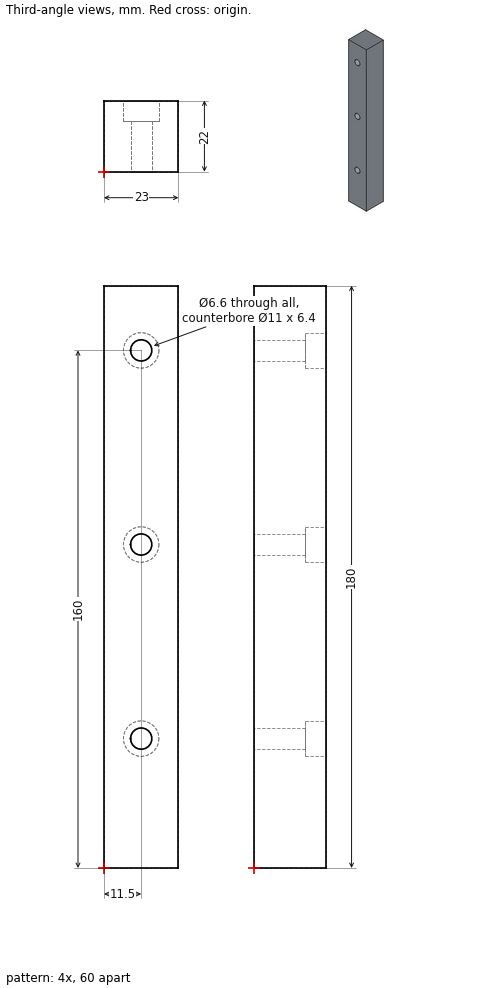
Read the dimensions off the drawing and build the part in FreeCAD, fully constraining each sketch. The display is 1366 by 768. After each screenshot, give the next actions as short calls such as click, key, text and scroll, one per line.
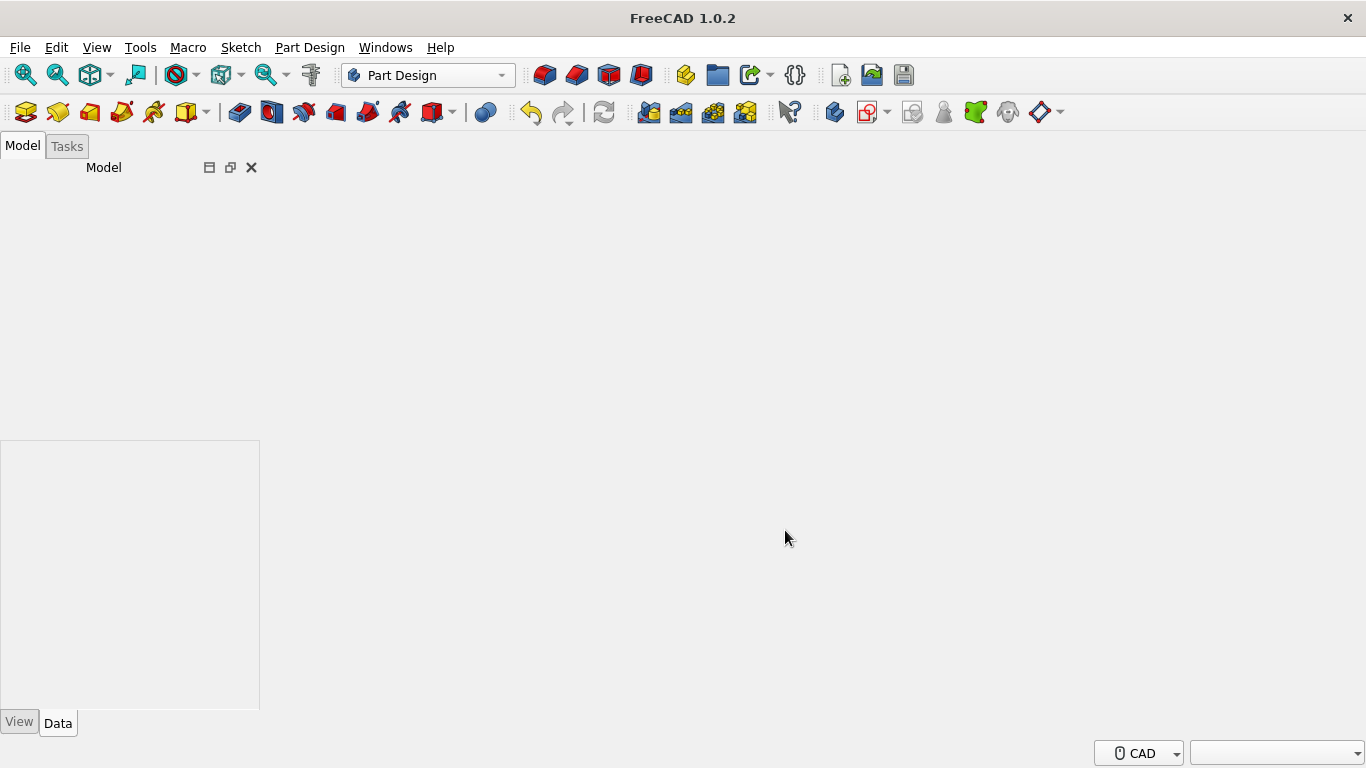
click(840, 76)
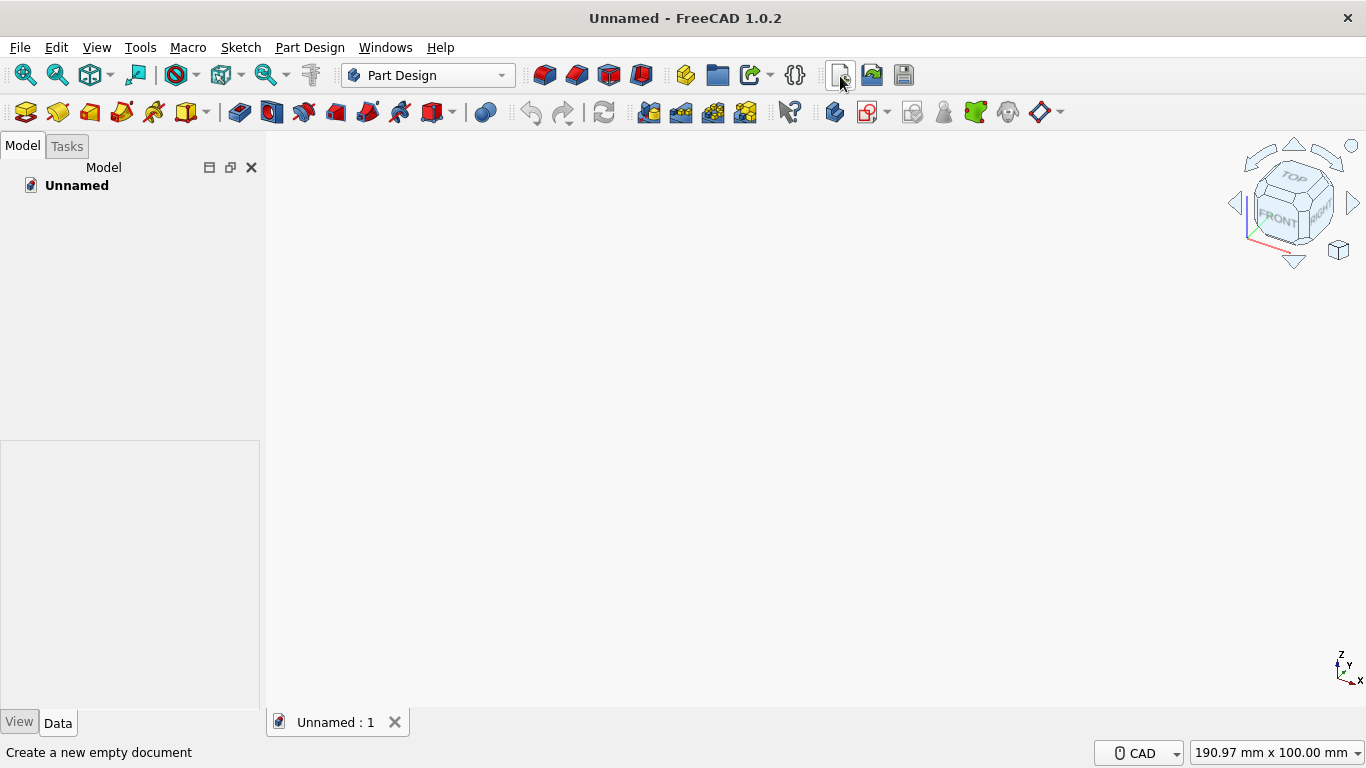
click(868, 112)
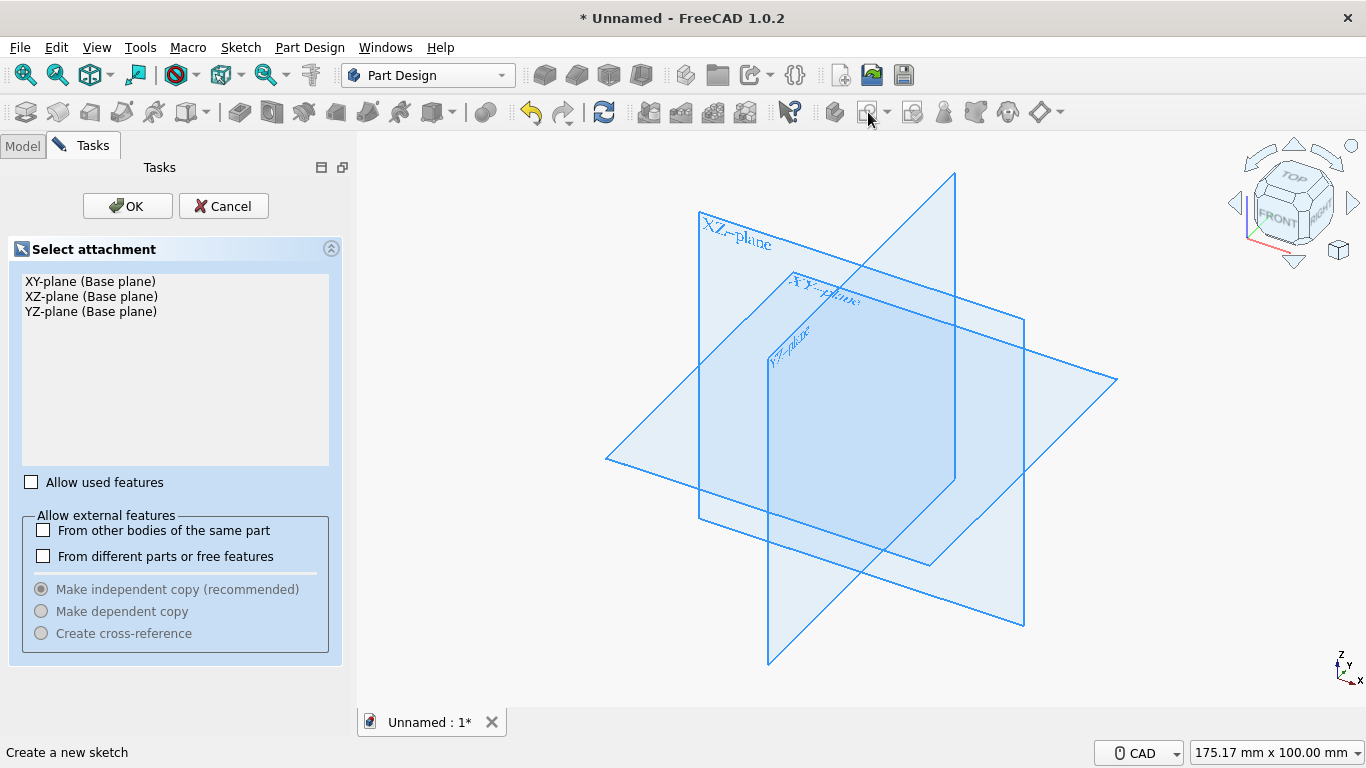
click(82, 282)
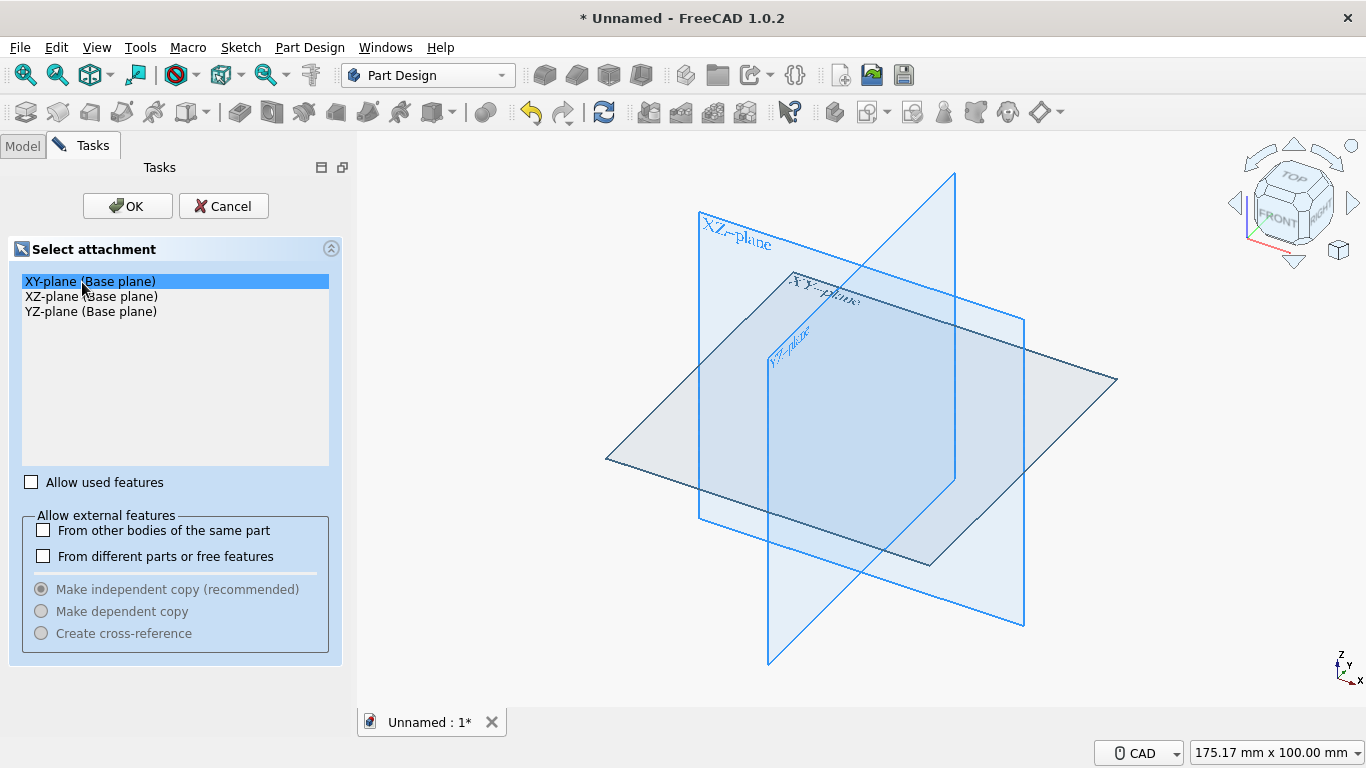
click(128, 206)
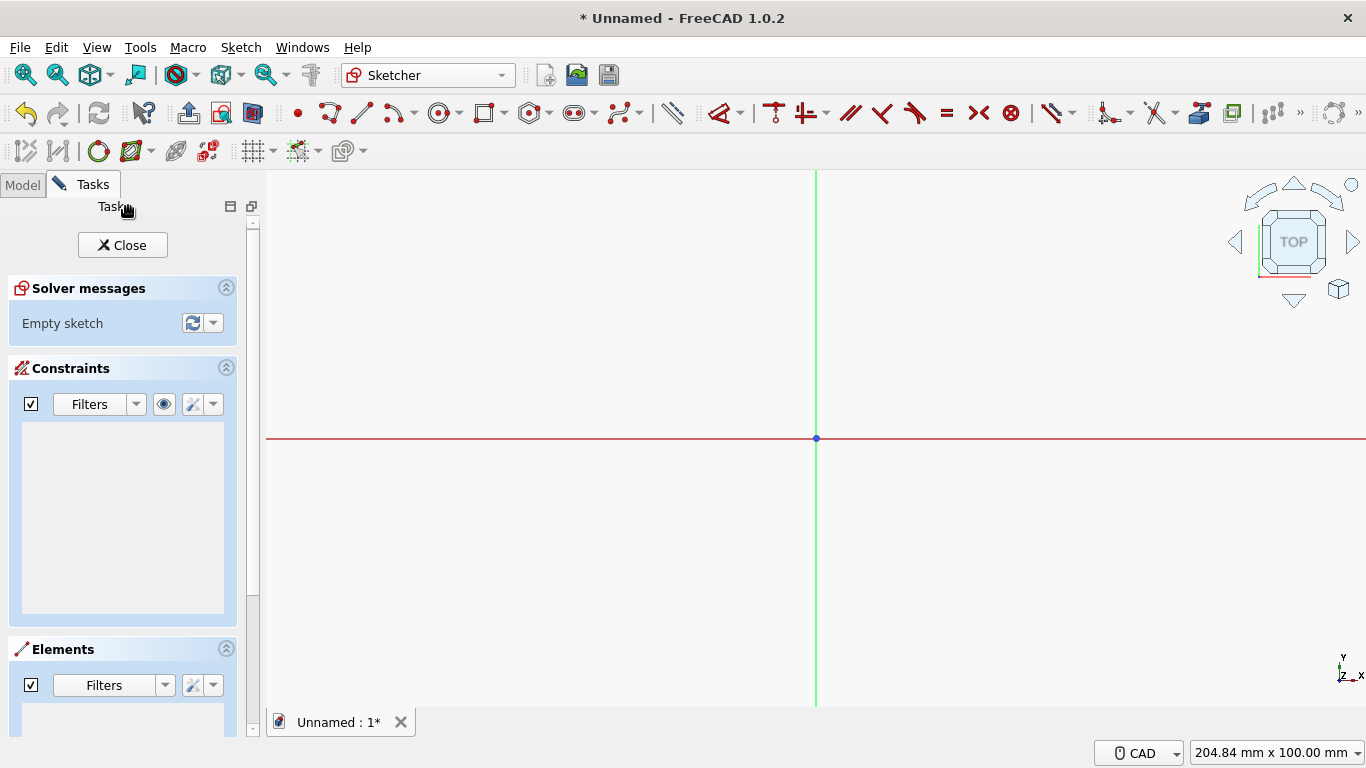
scroll(954, 345, up, 5)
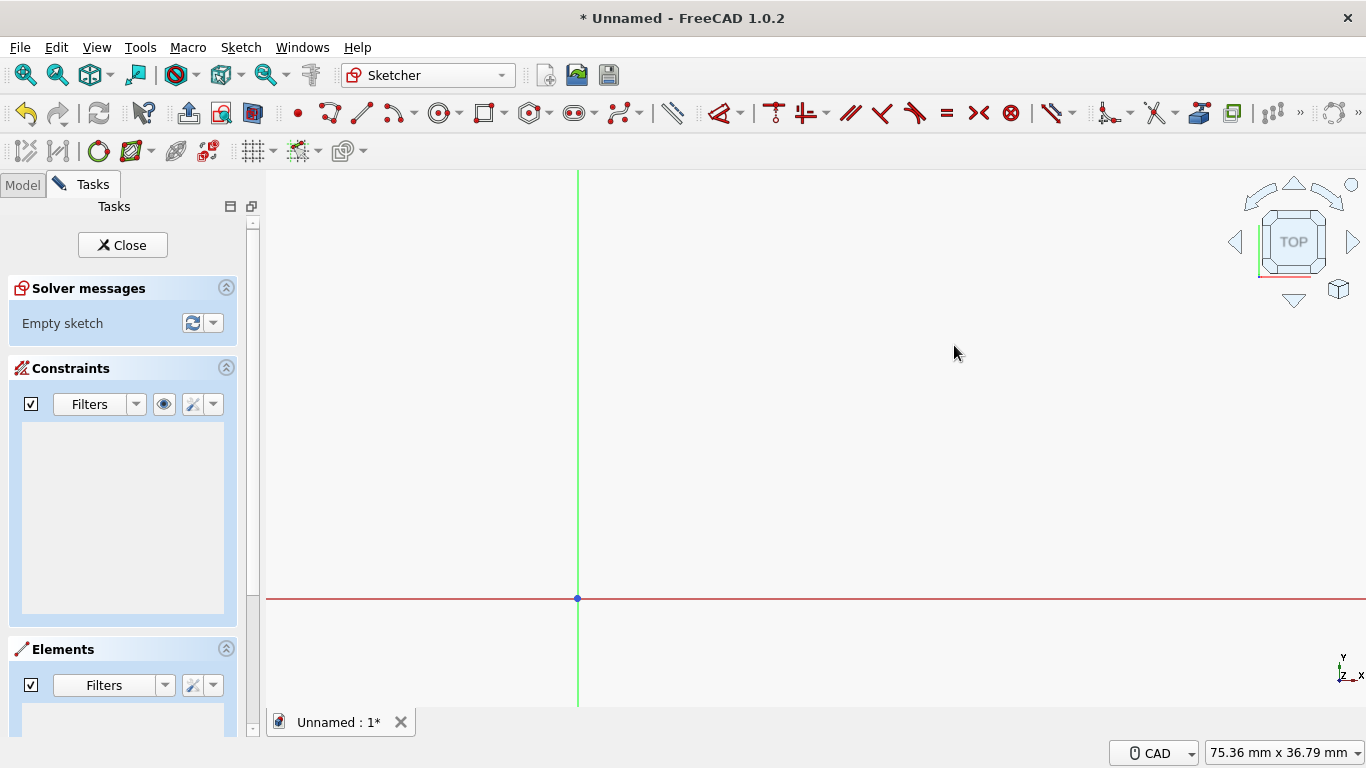
click(484, 114)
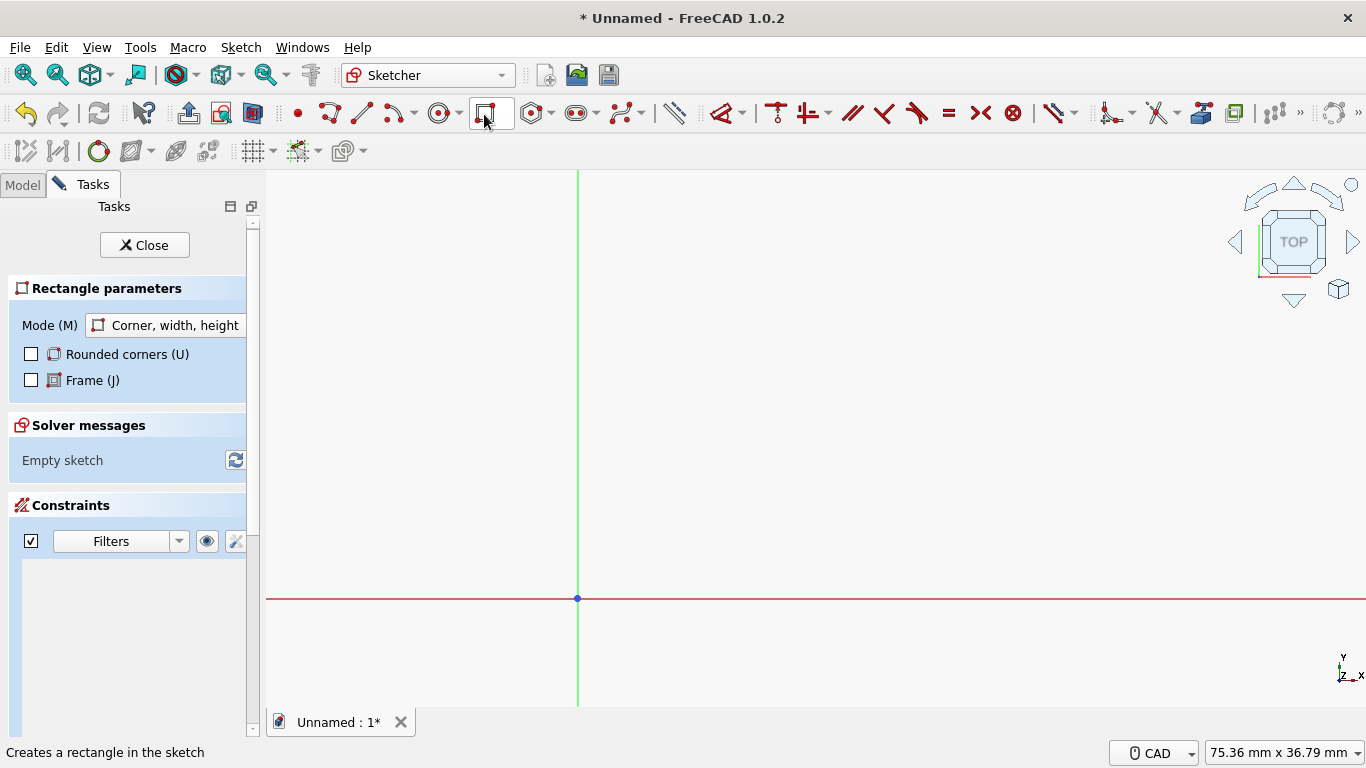
click(578, 599)
click(914, 277)
key(Escape)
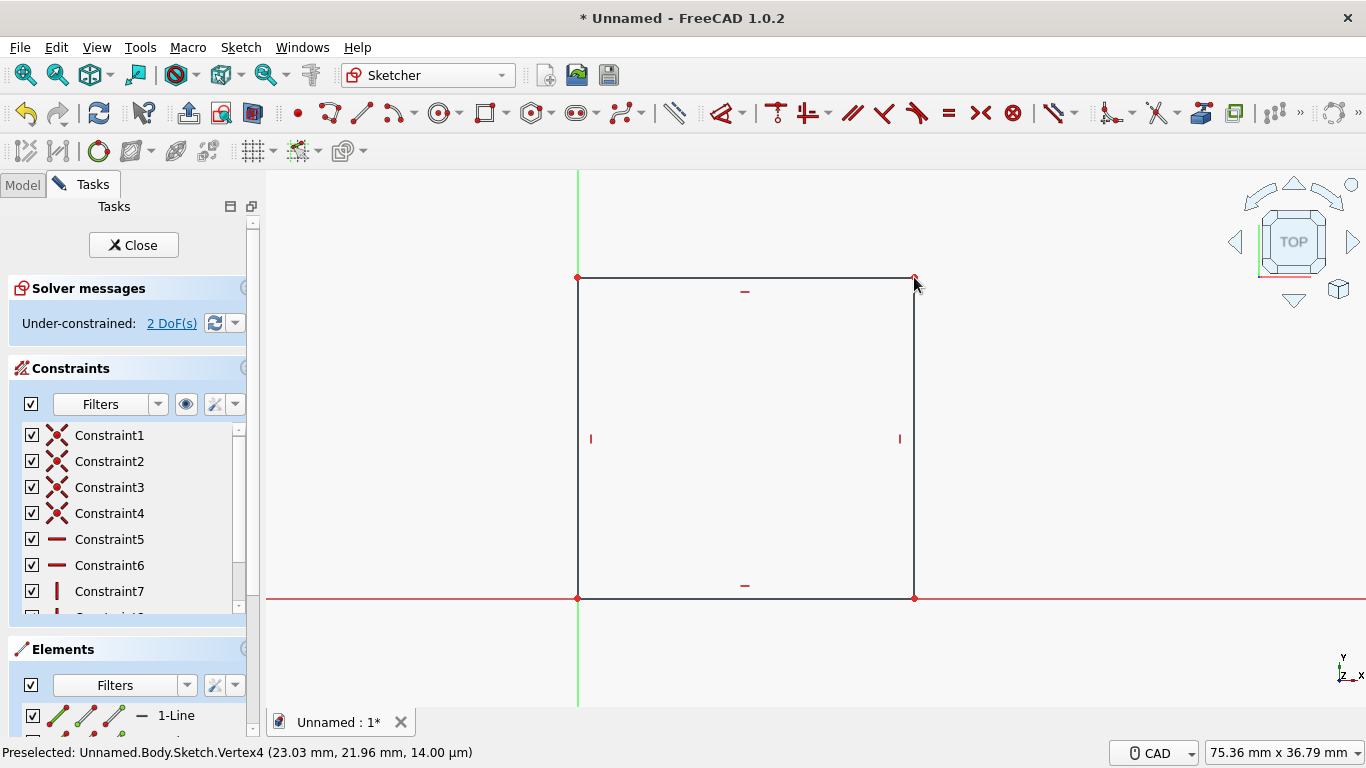
click(679, 599)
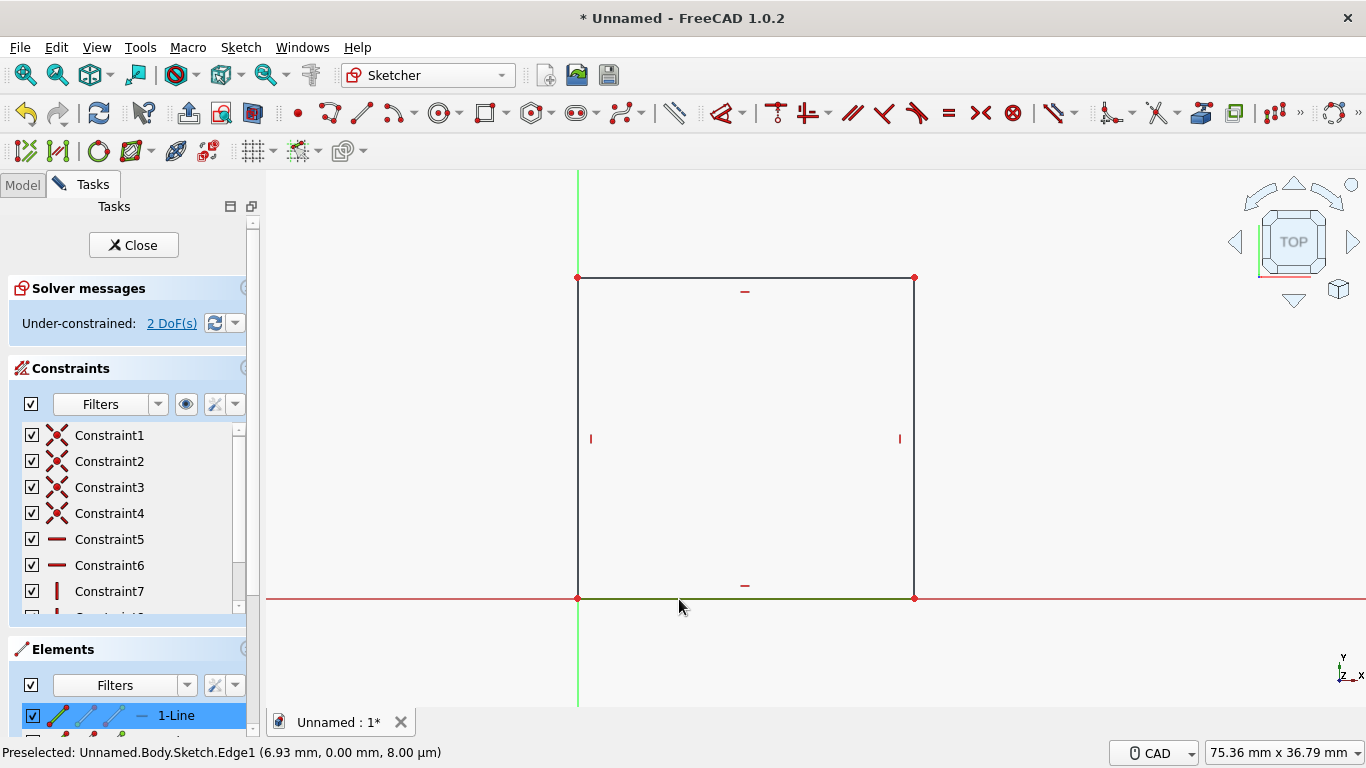
key(l)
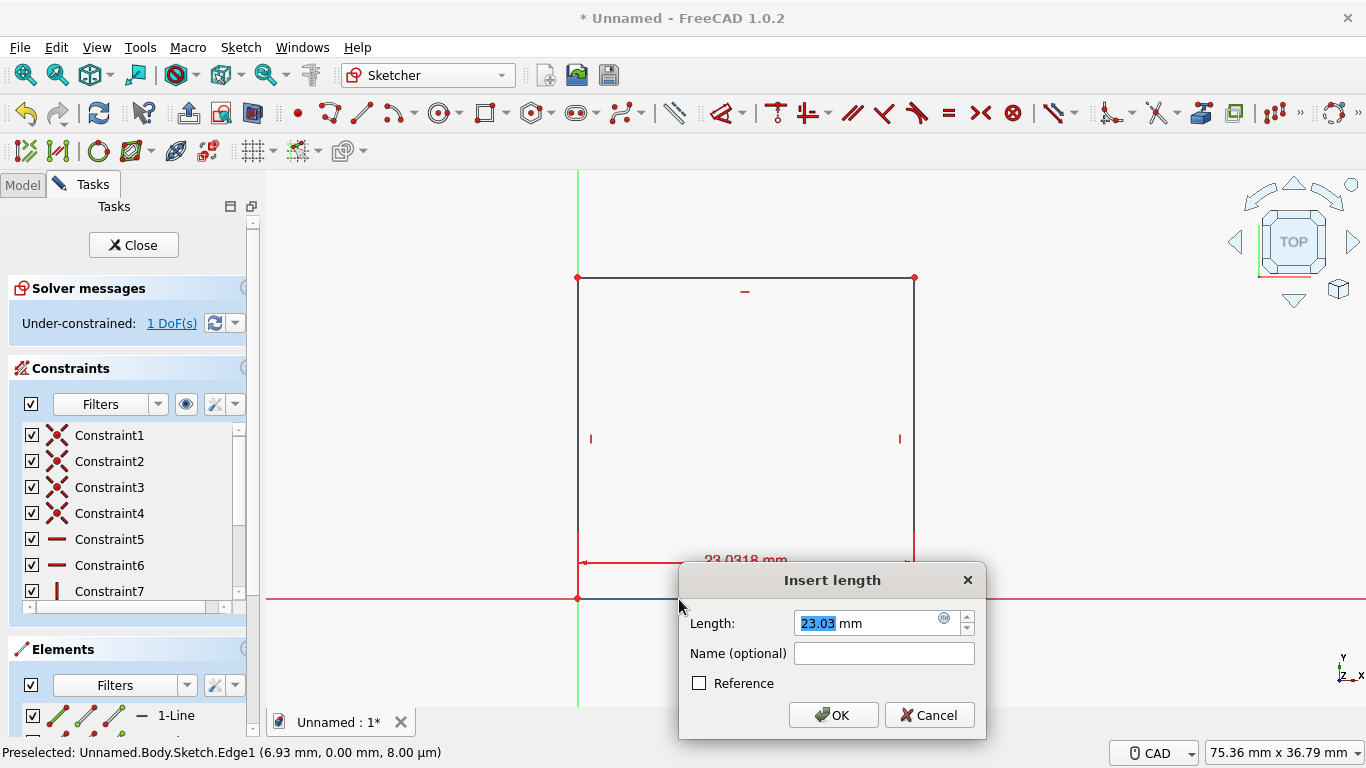
text(23)
key(Return)